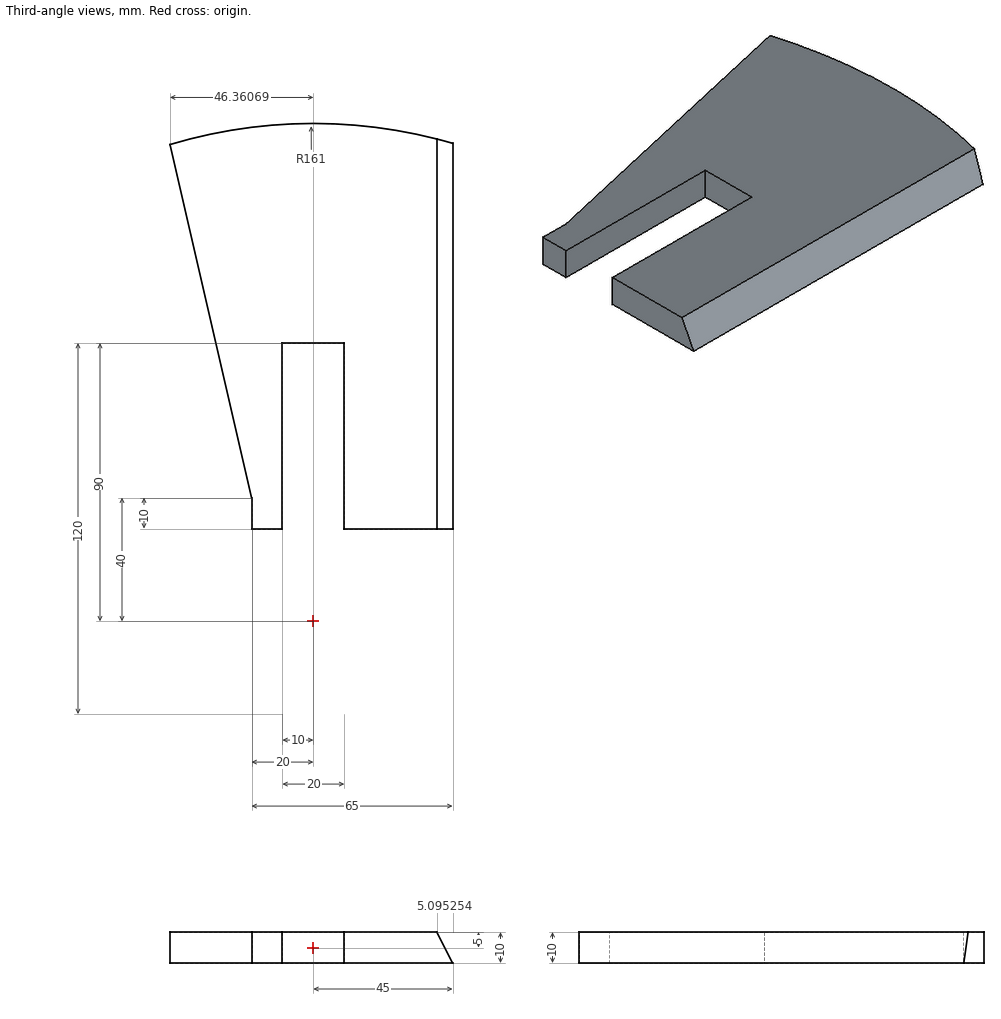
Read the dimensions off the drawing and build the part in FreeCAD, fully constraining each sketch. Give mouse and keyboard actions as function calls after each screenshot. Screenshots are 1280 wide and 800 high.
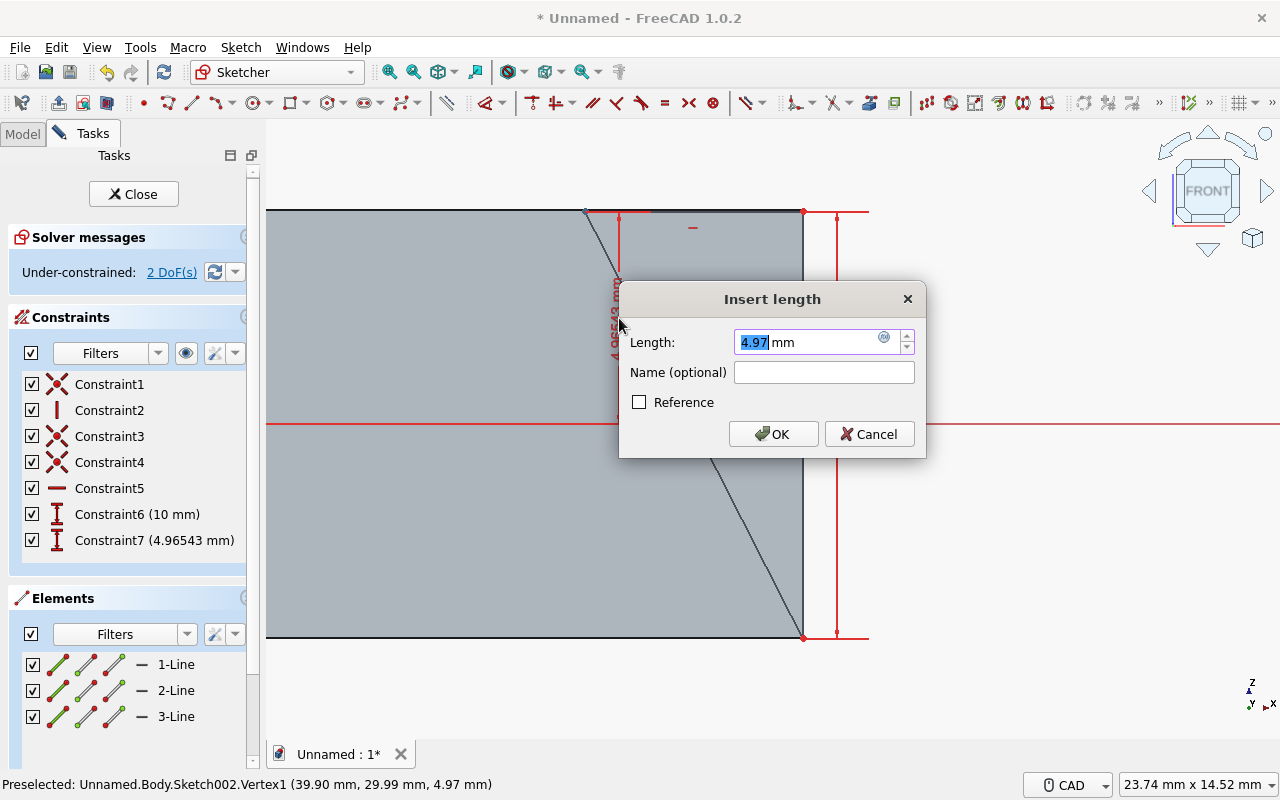
text(5)
key(Return)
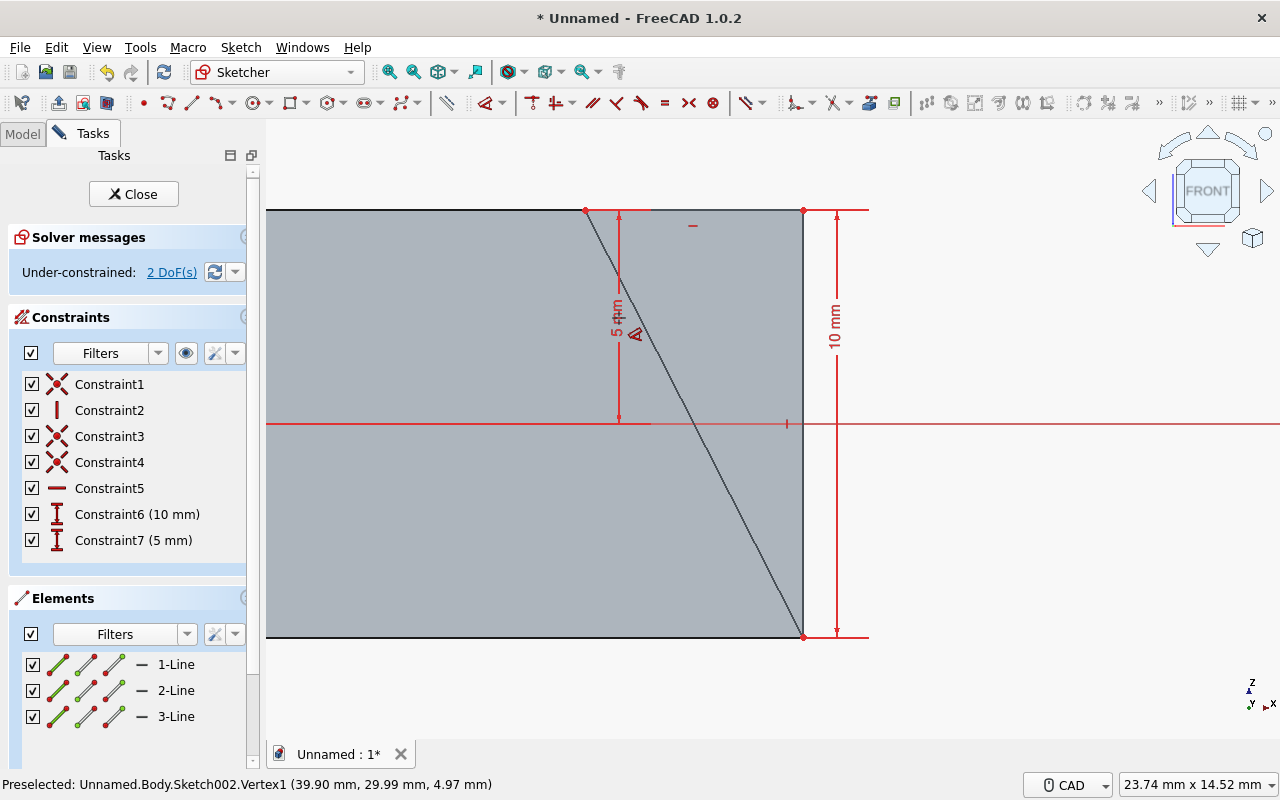
click(803, 638)
click(549, 672)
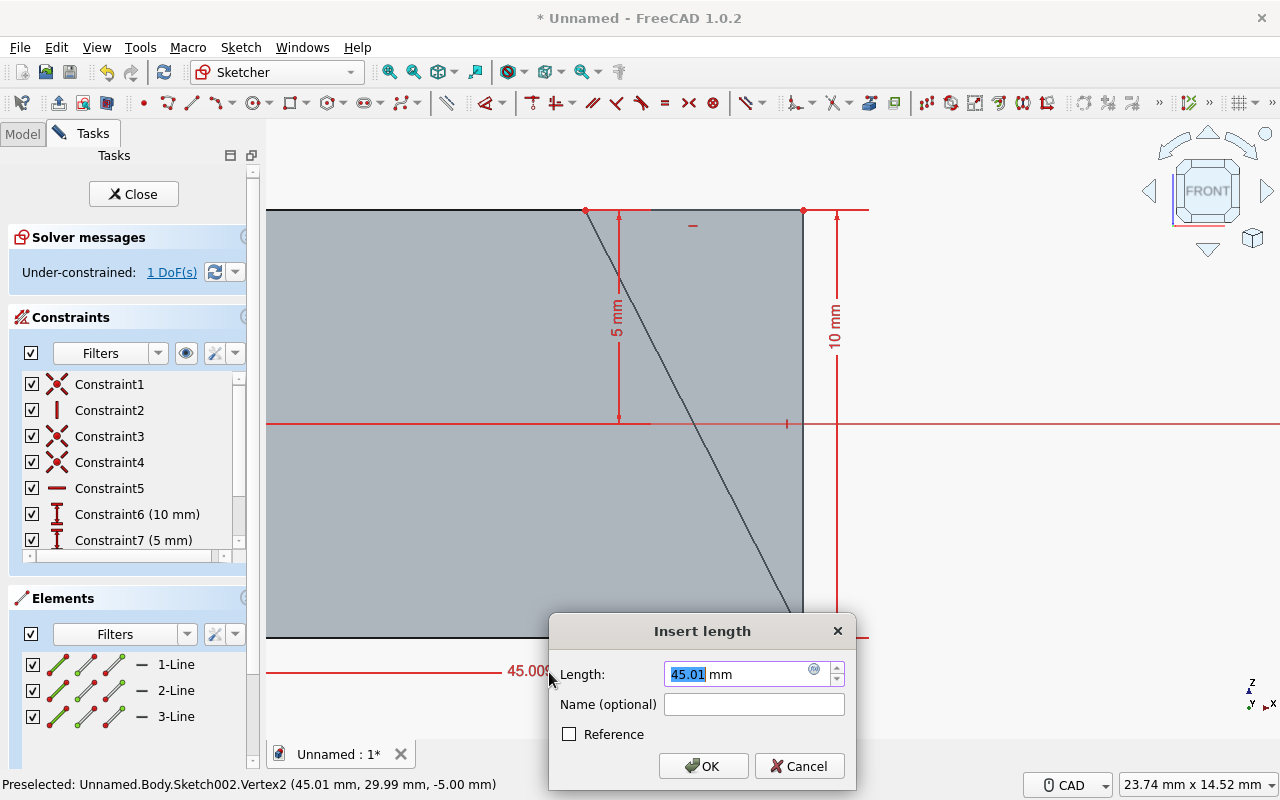
text(45)
key(Return)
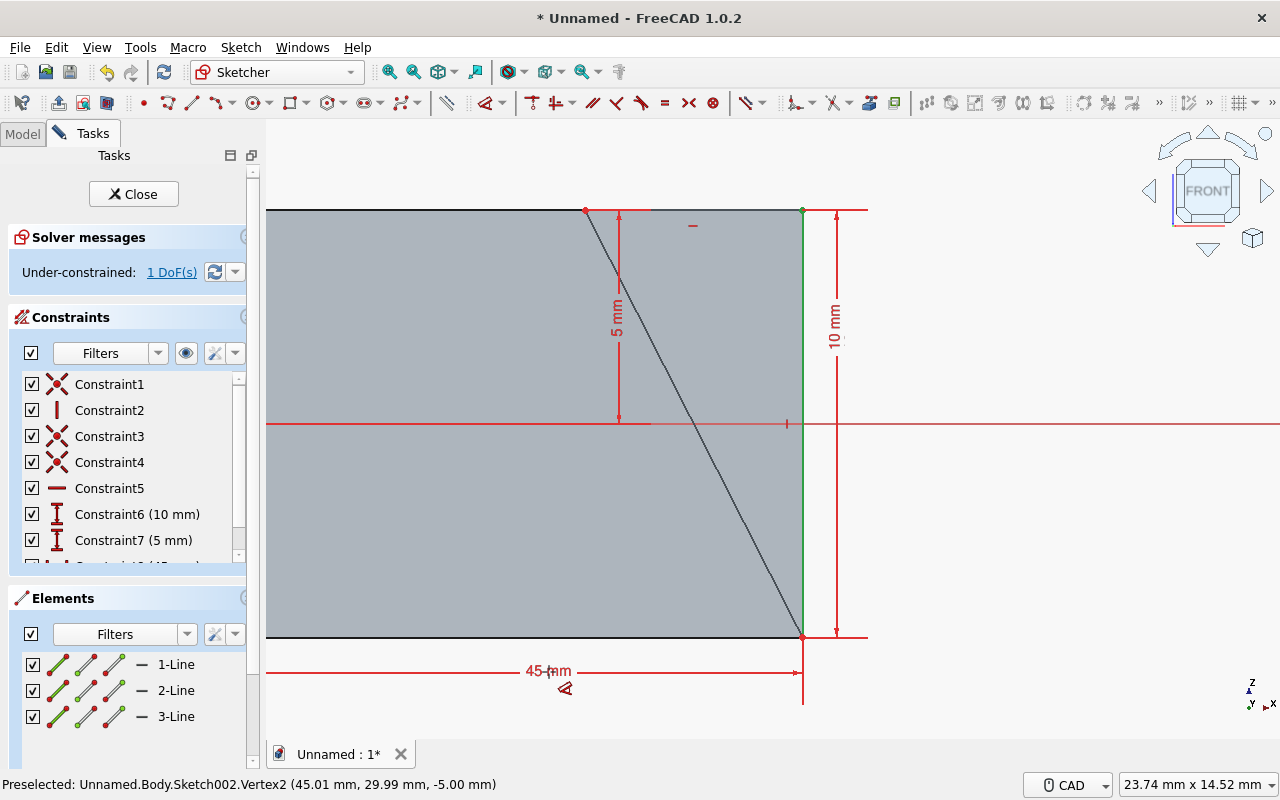
click(737, 210)
click(694, 176)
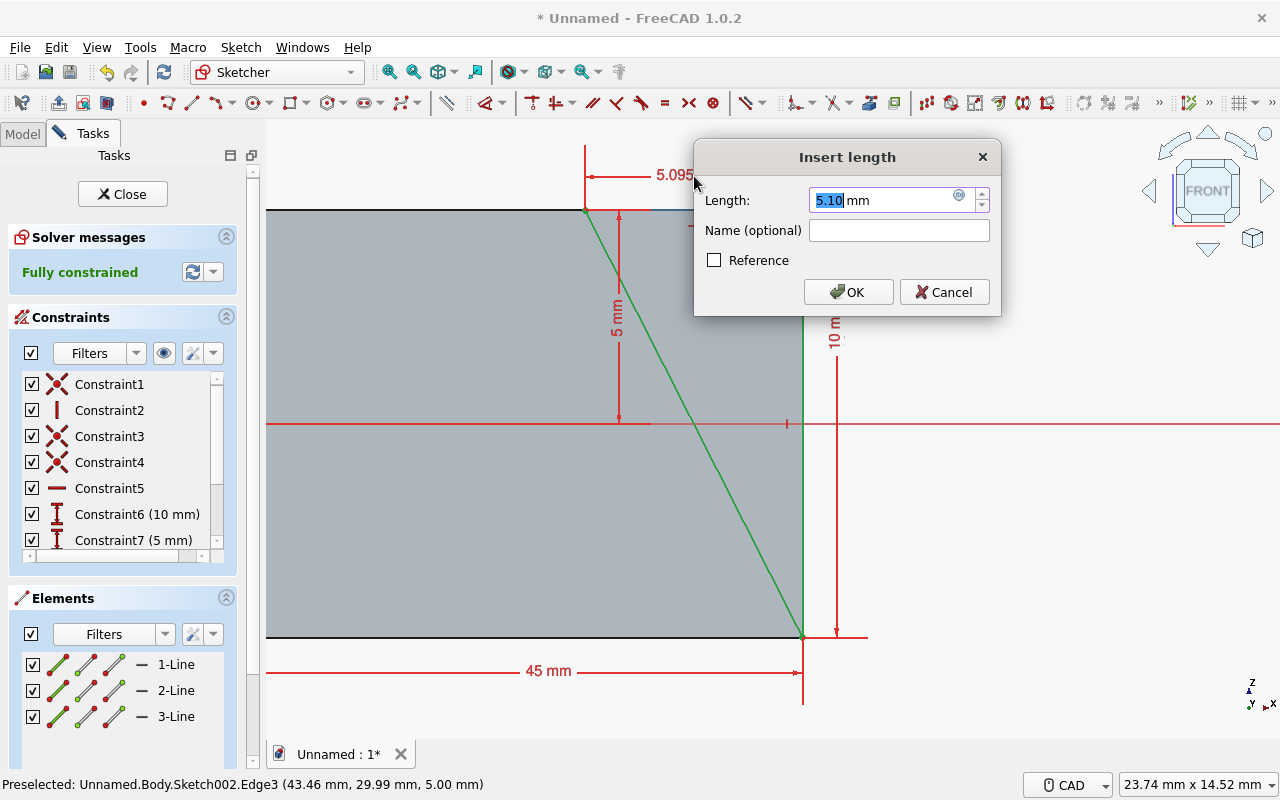
text(5.095254)
key(Return)
key(Escape)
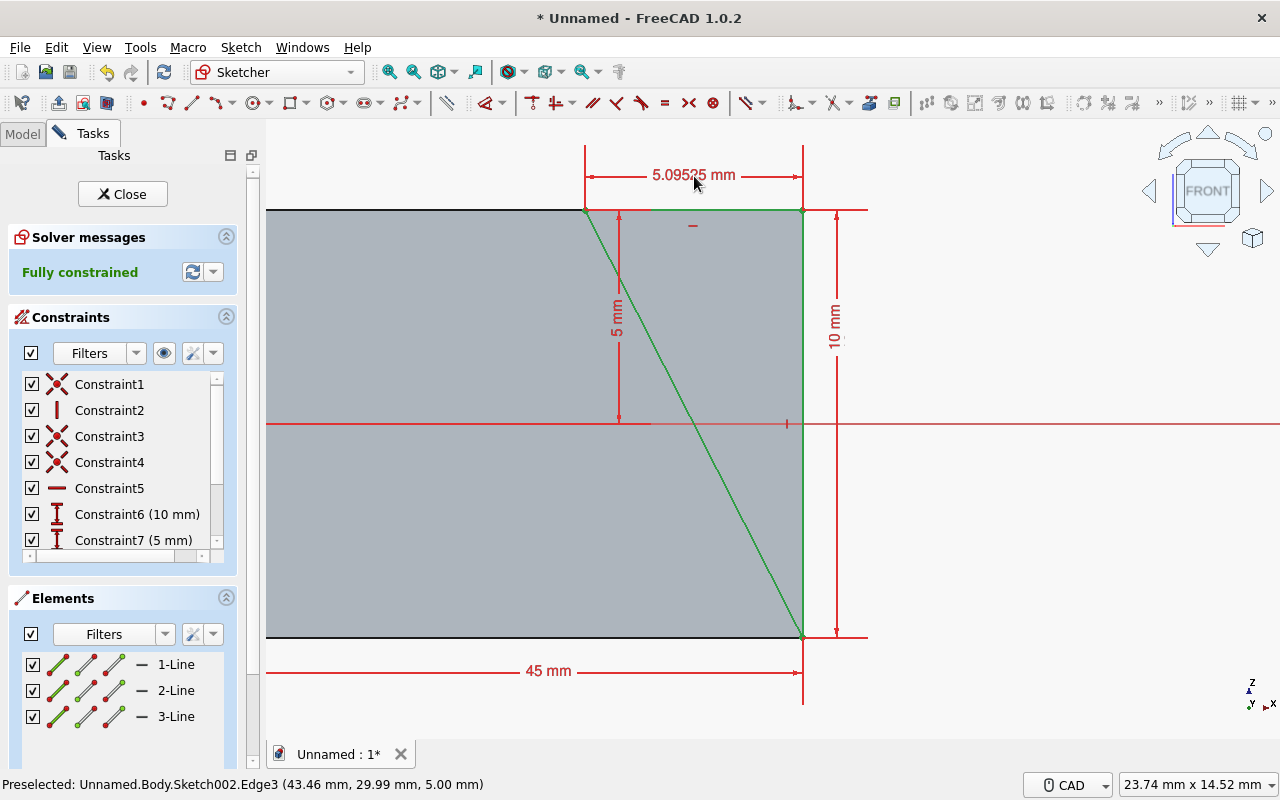
click(123, 194)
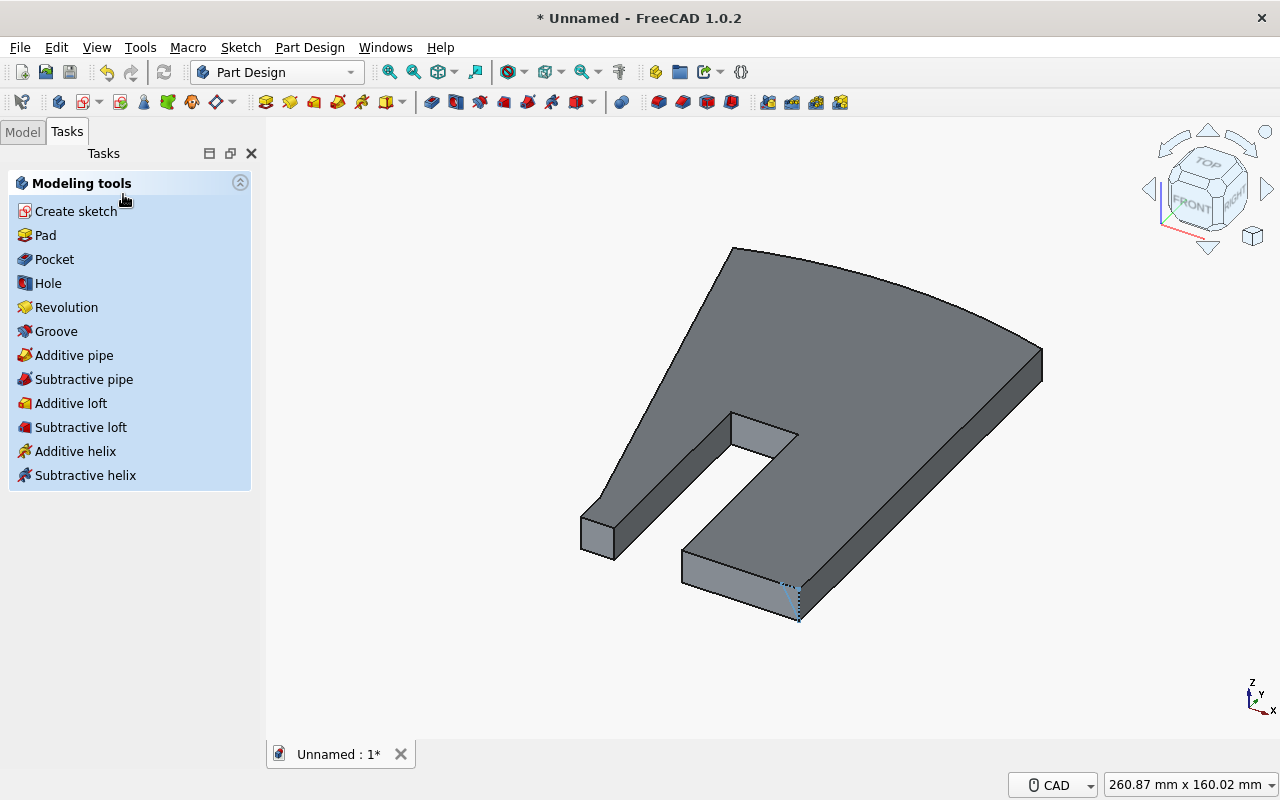
click(432, 102)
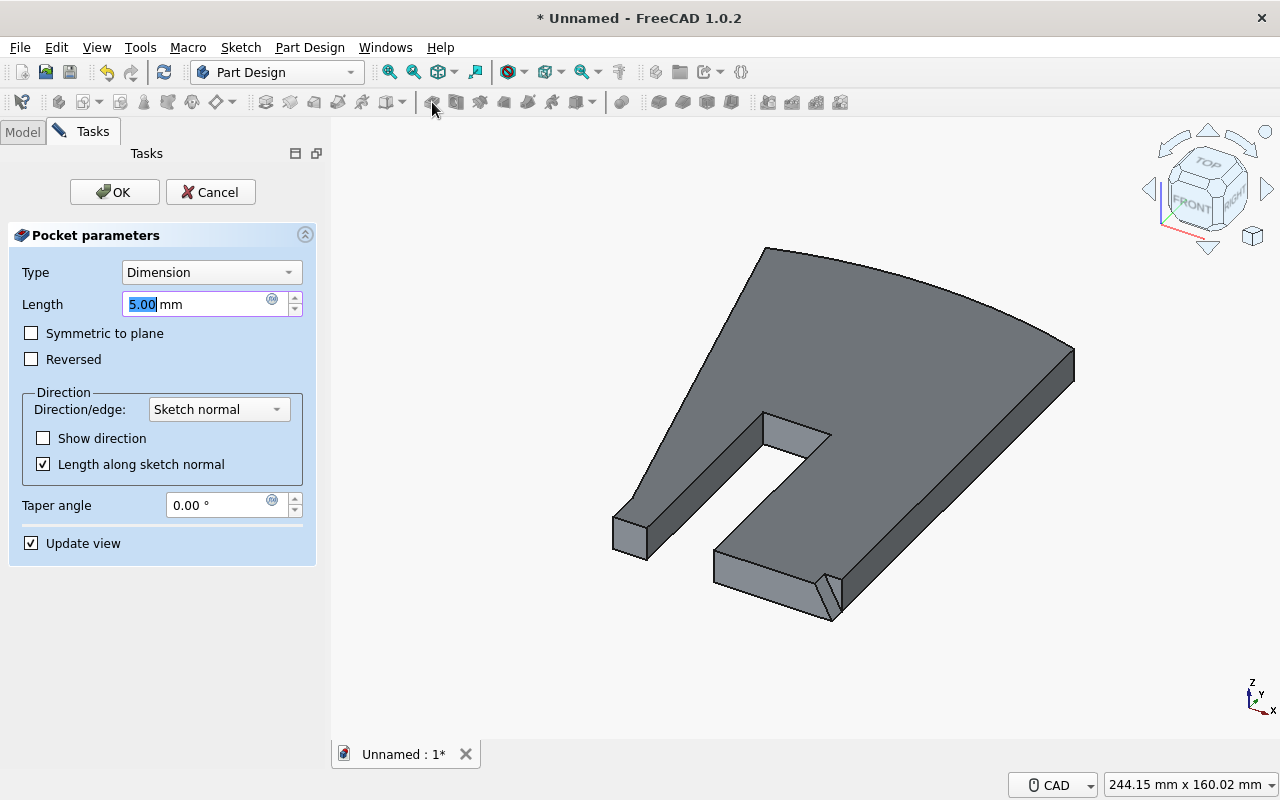
click(212, 272)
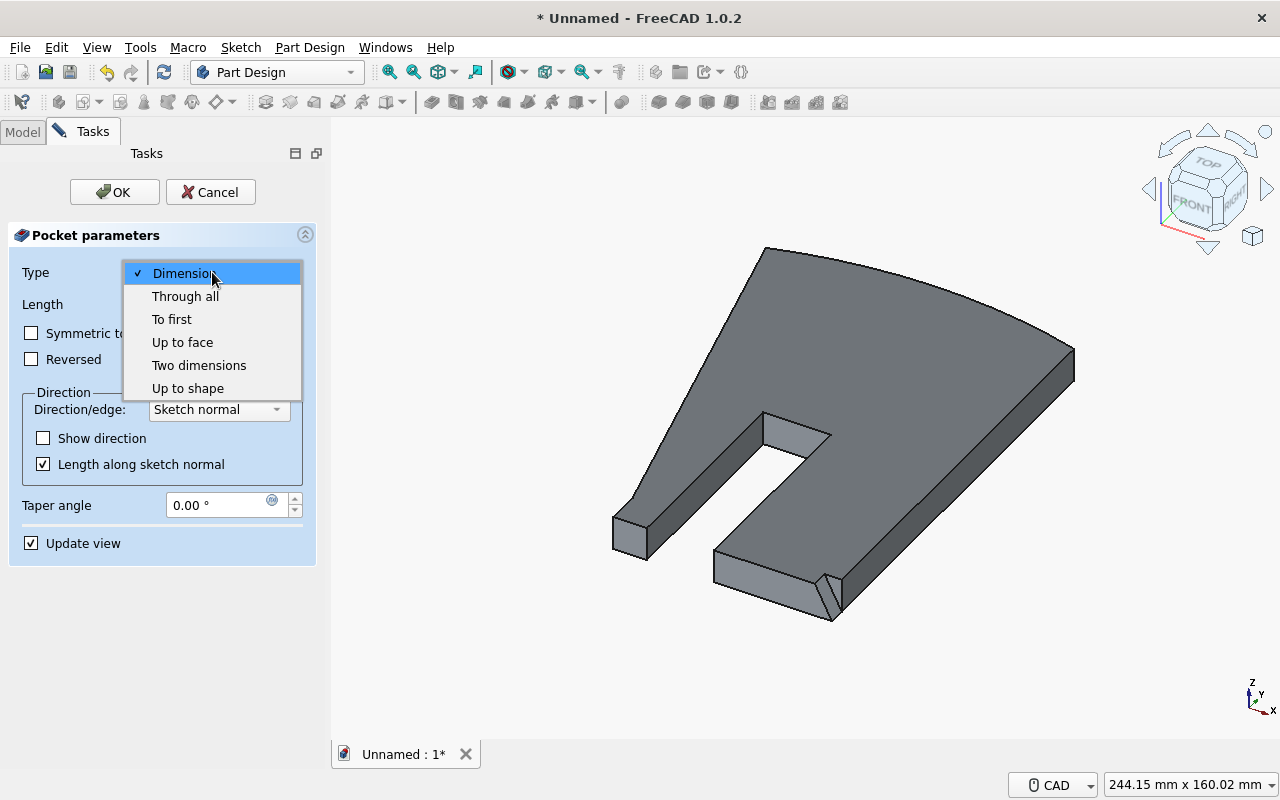
click(212, 296)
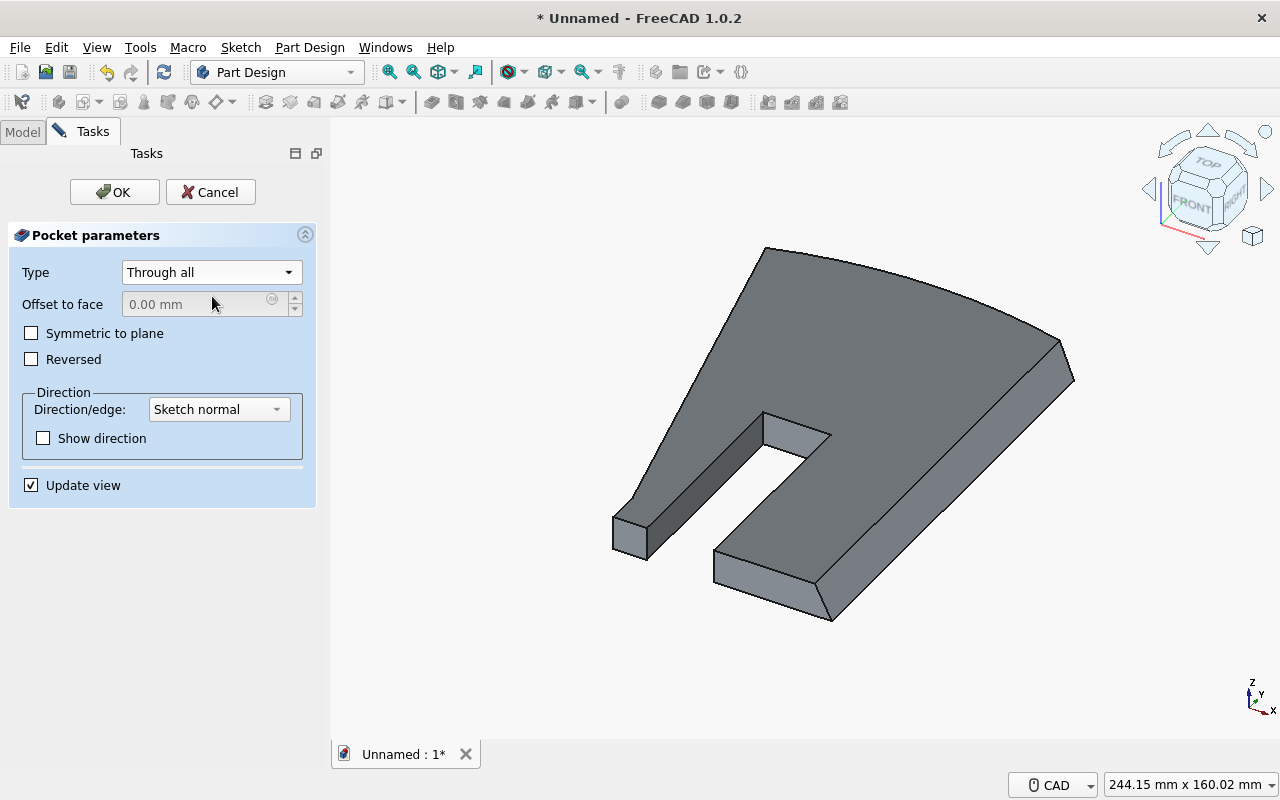
click(115, 192)